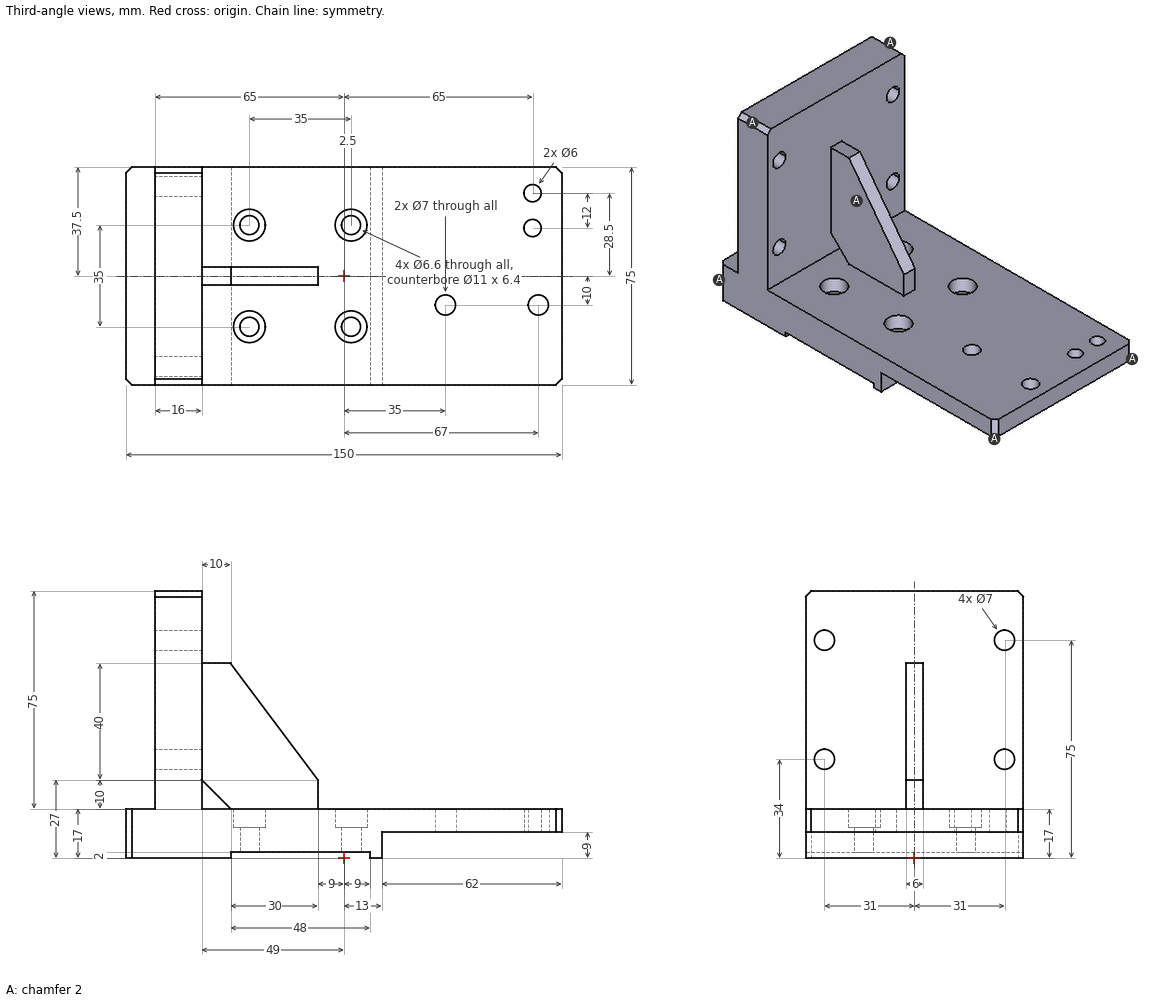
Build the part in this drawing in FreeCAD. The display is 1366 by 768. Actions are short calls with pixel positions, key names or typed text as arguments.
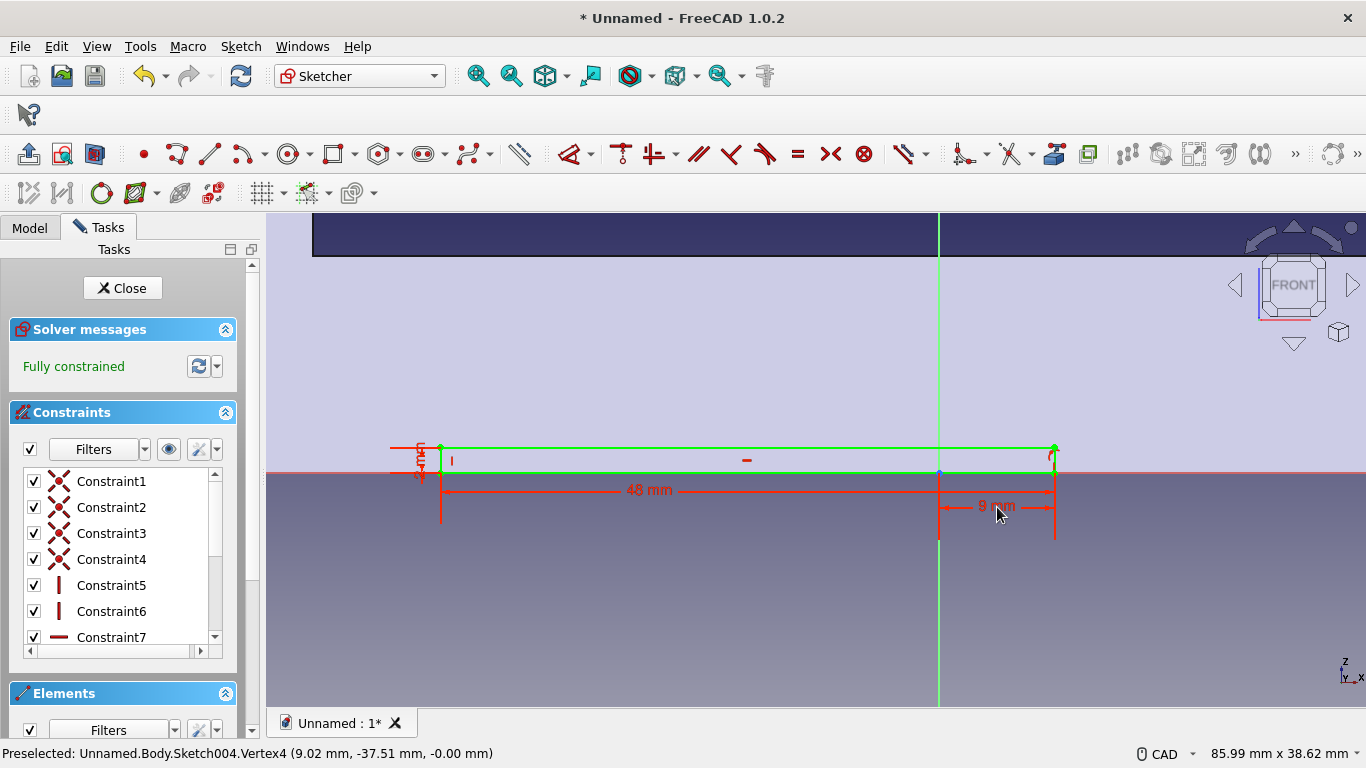
click(123, 288)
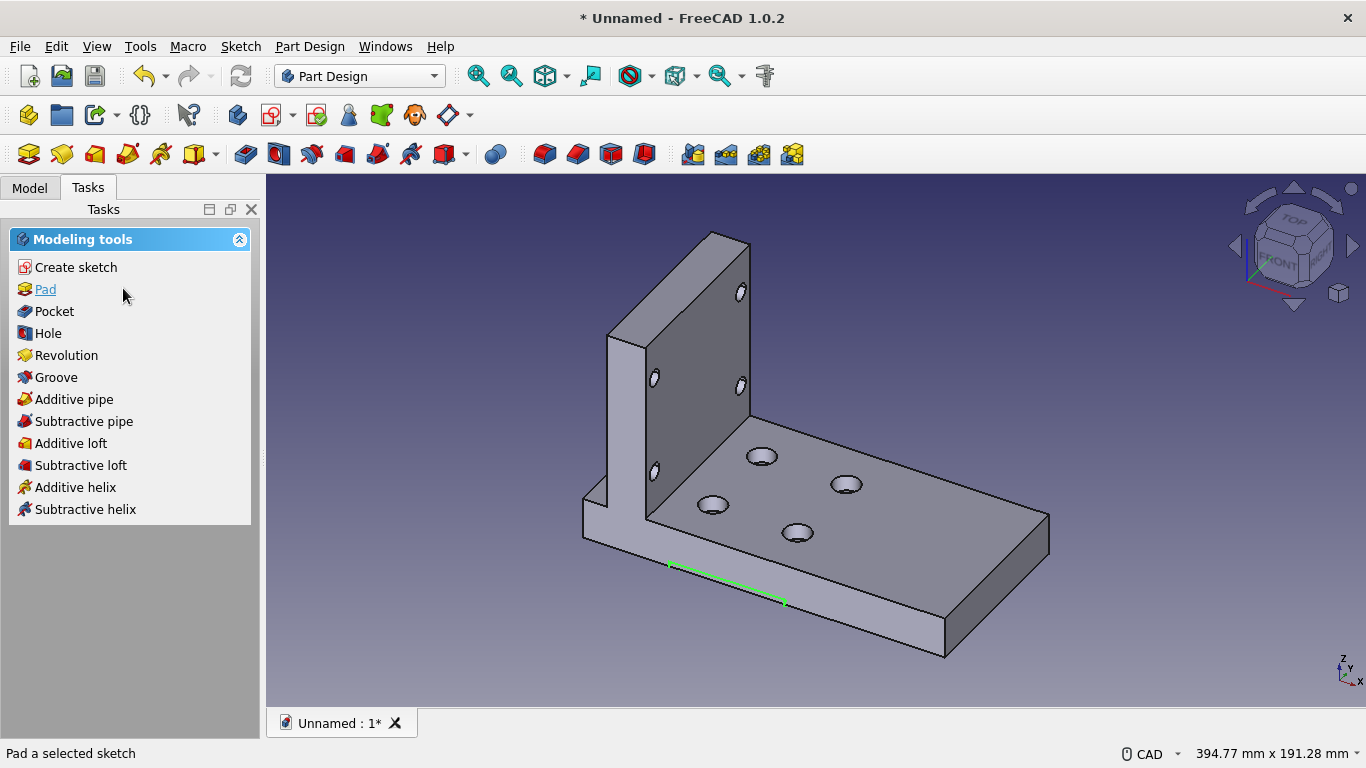
click(246, 154)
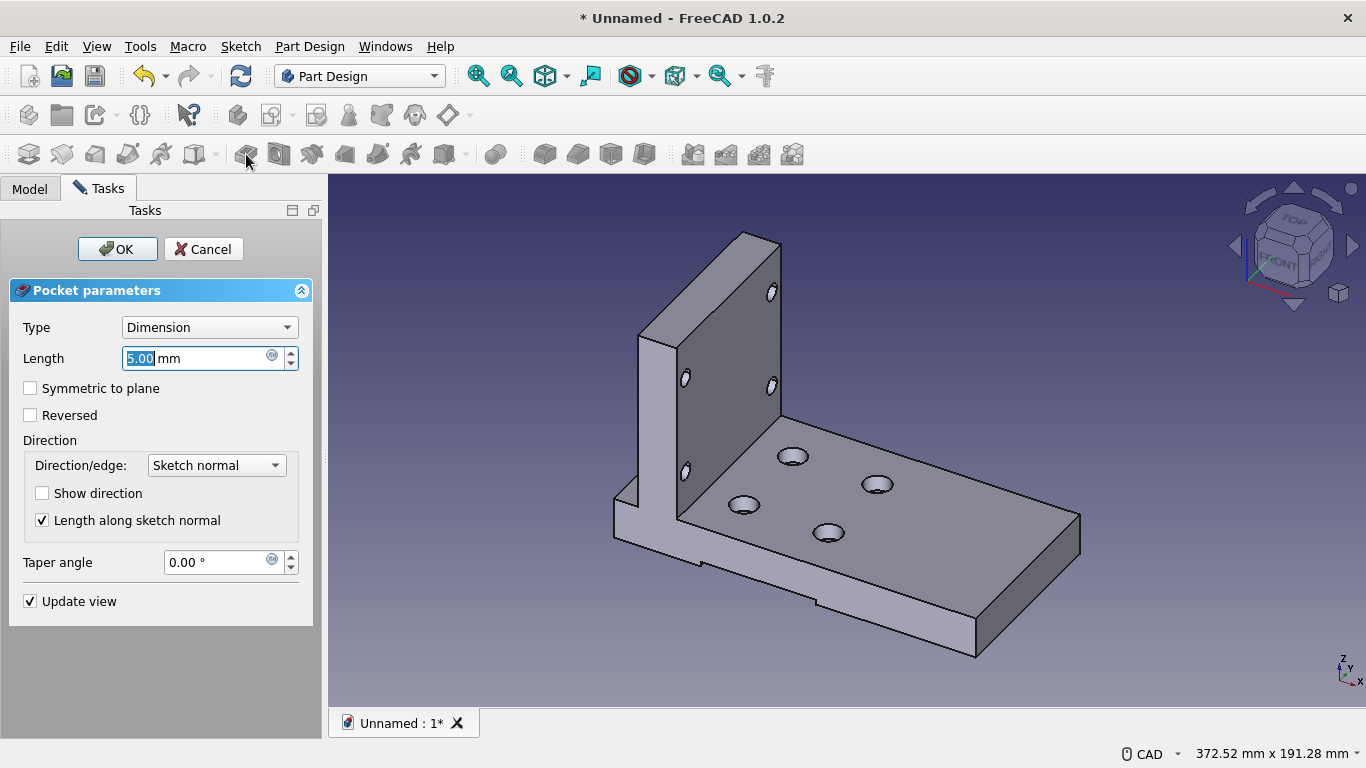
click(210, 328)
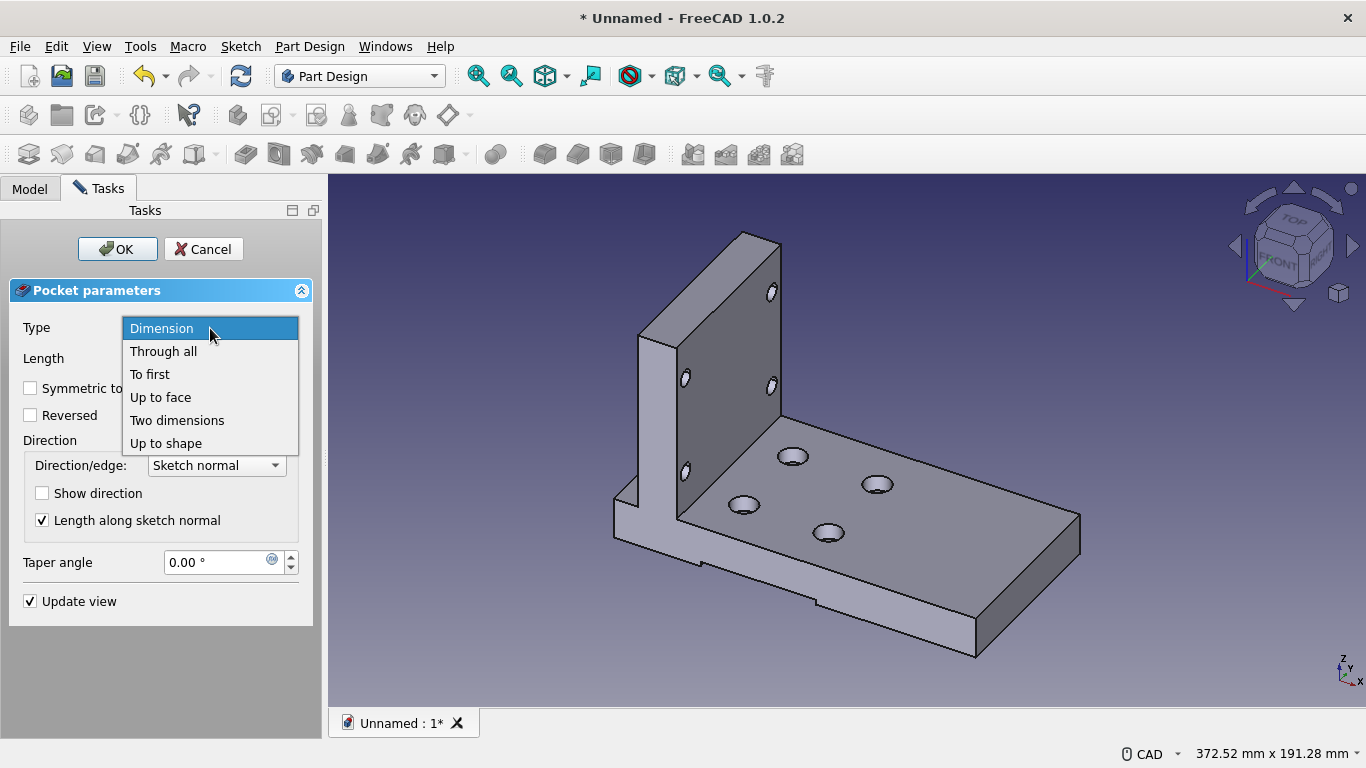
click(208, 352)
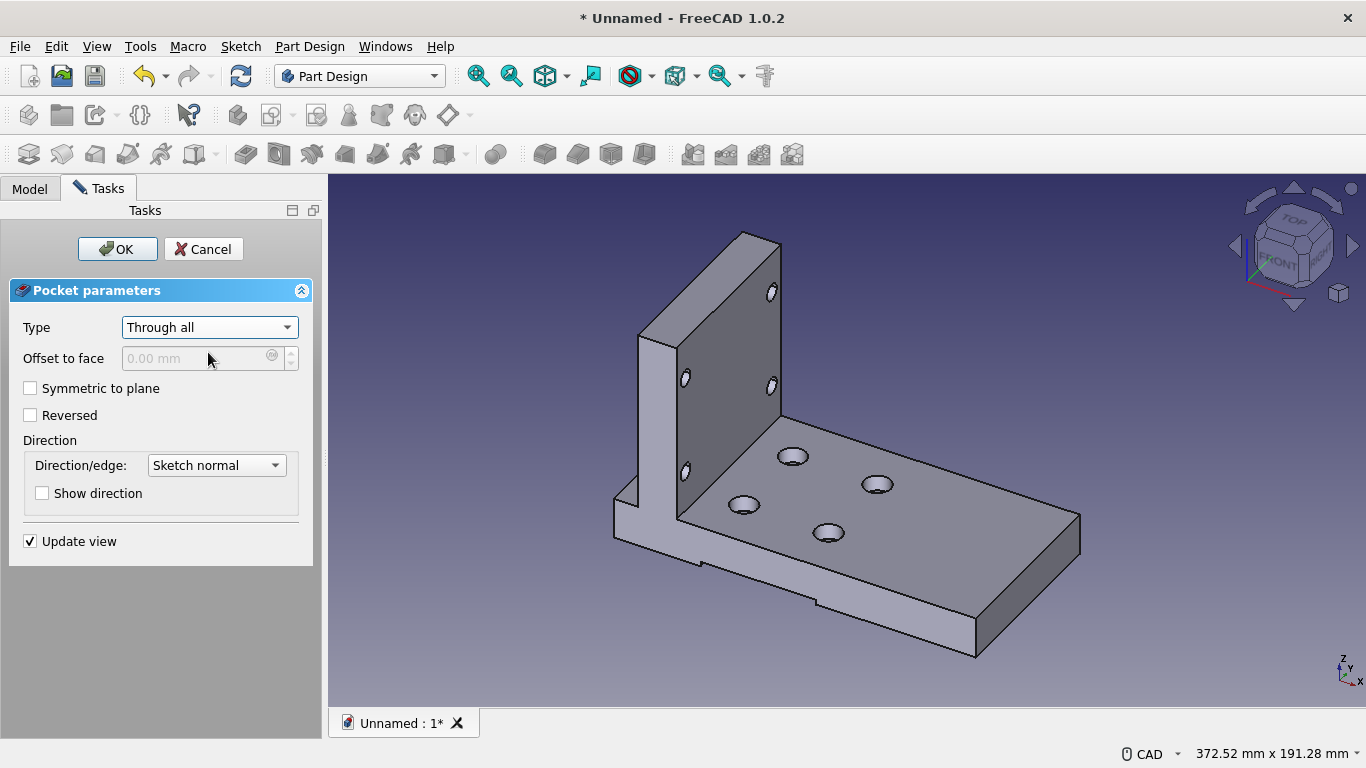
click(118, 249)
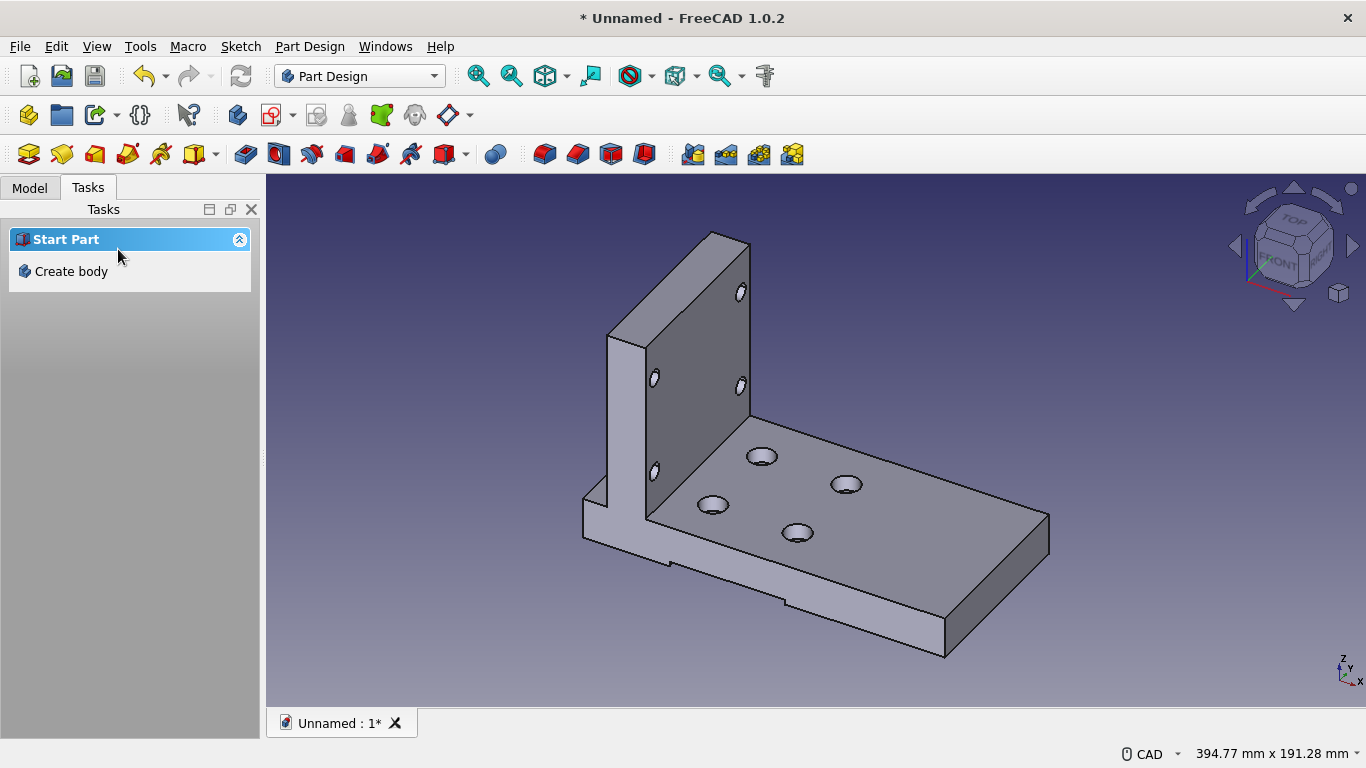
click(270, 116)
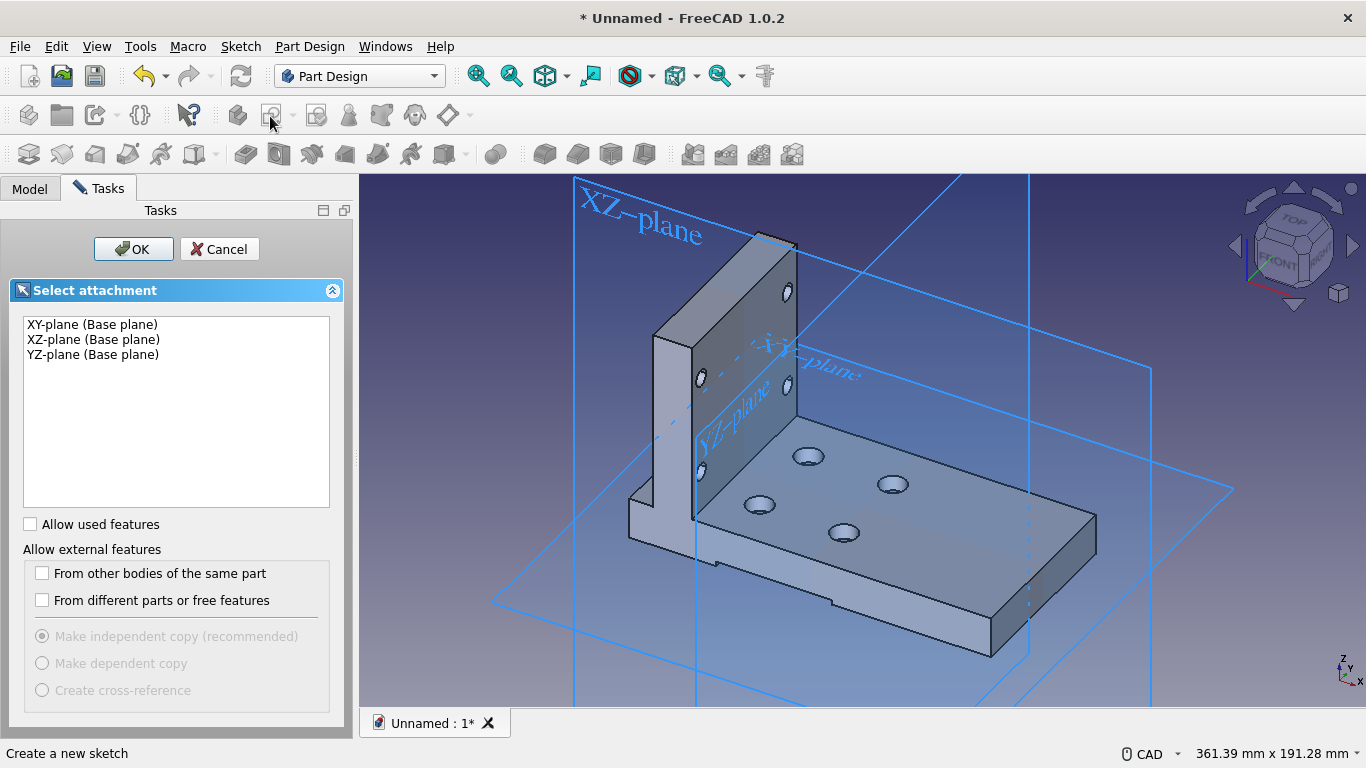
click(84, 340)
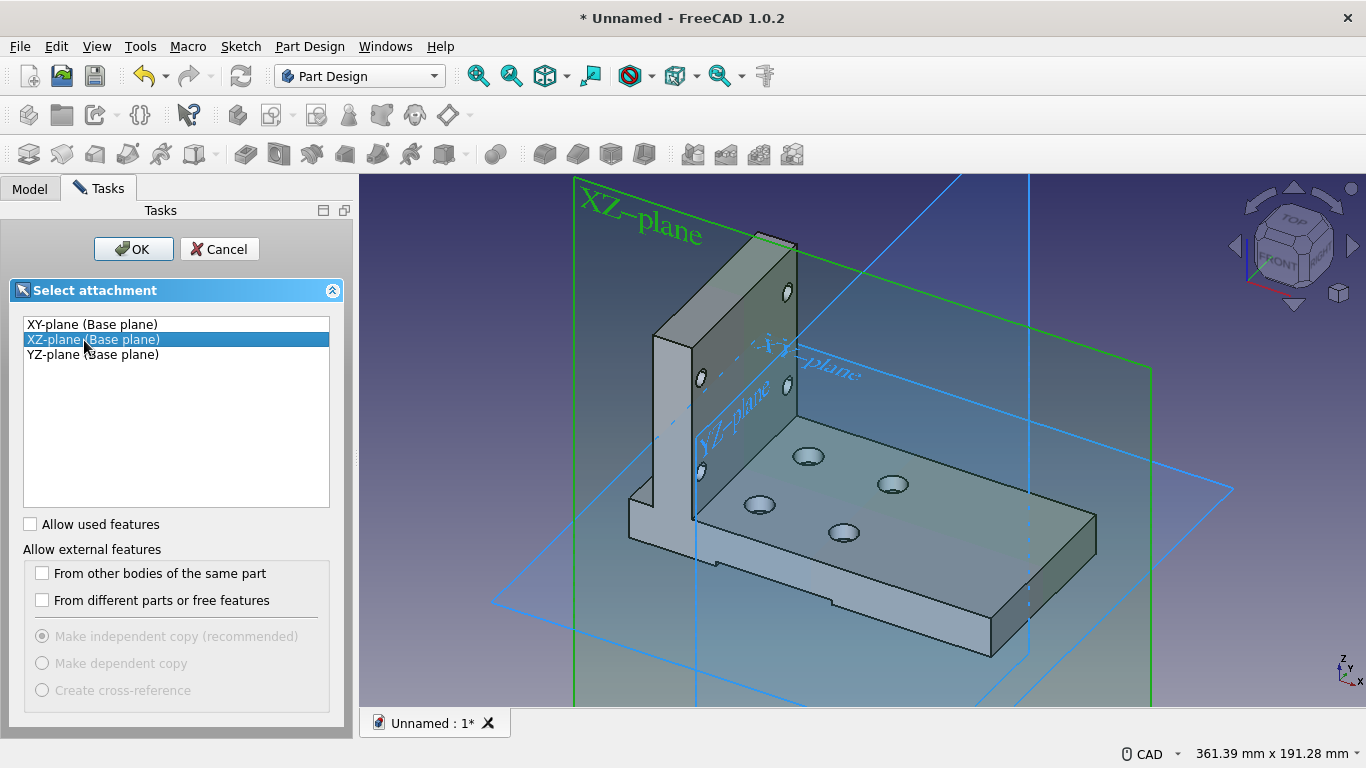
click(134, 249)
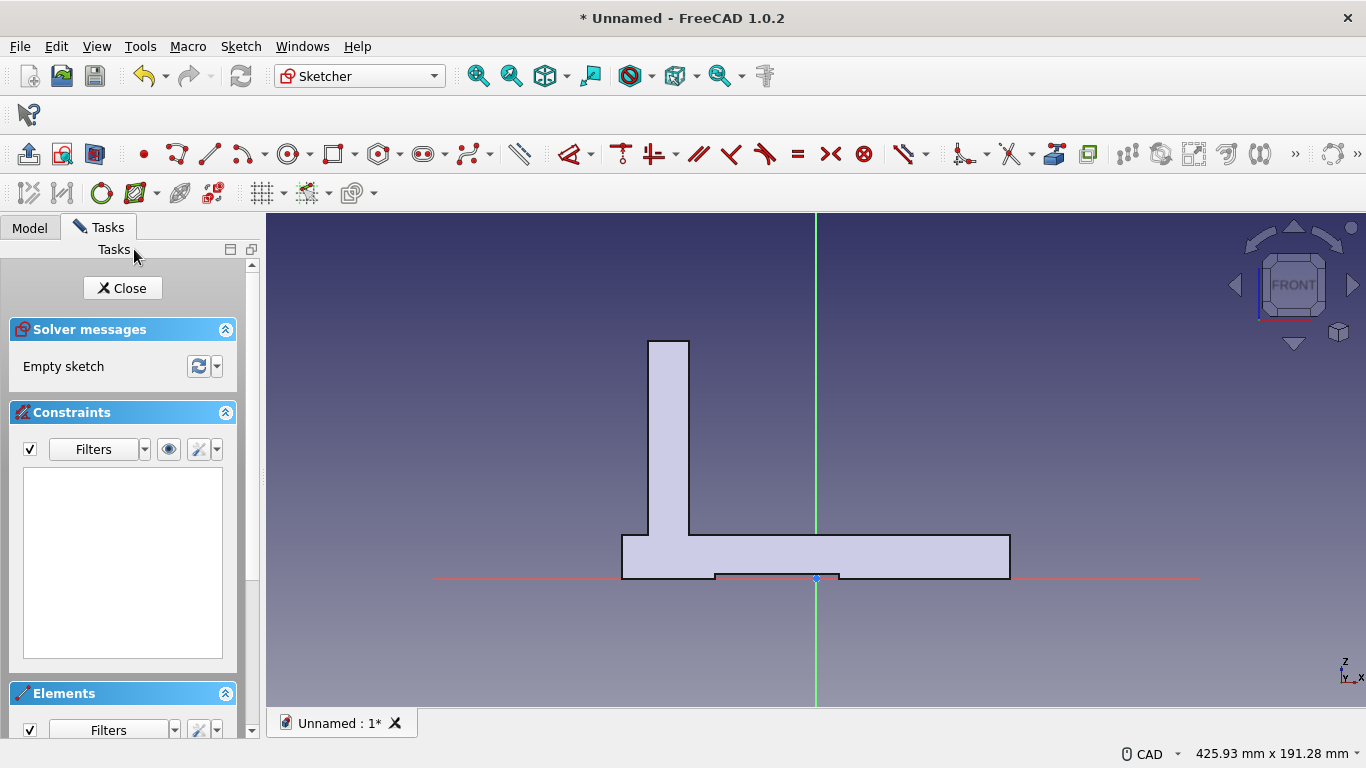
click(95, 154)